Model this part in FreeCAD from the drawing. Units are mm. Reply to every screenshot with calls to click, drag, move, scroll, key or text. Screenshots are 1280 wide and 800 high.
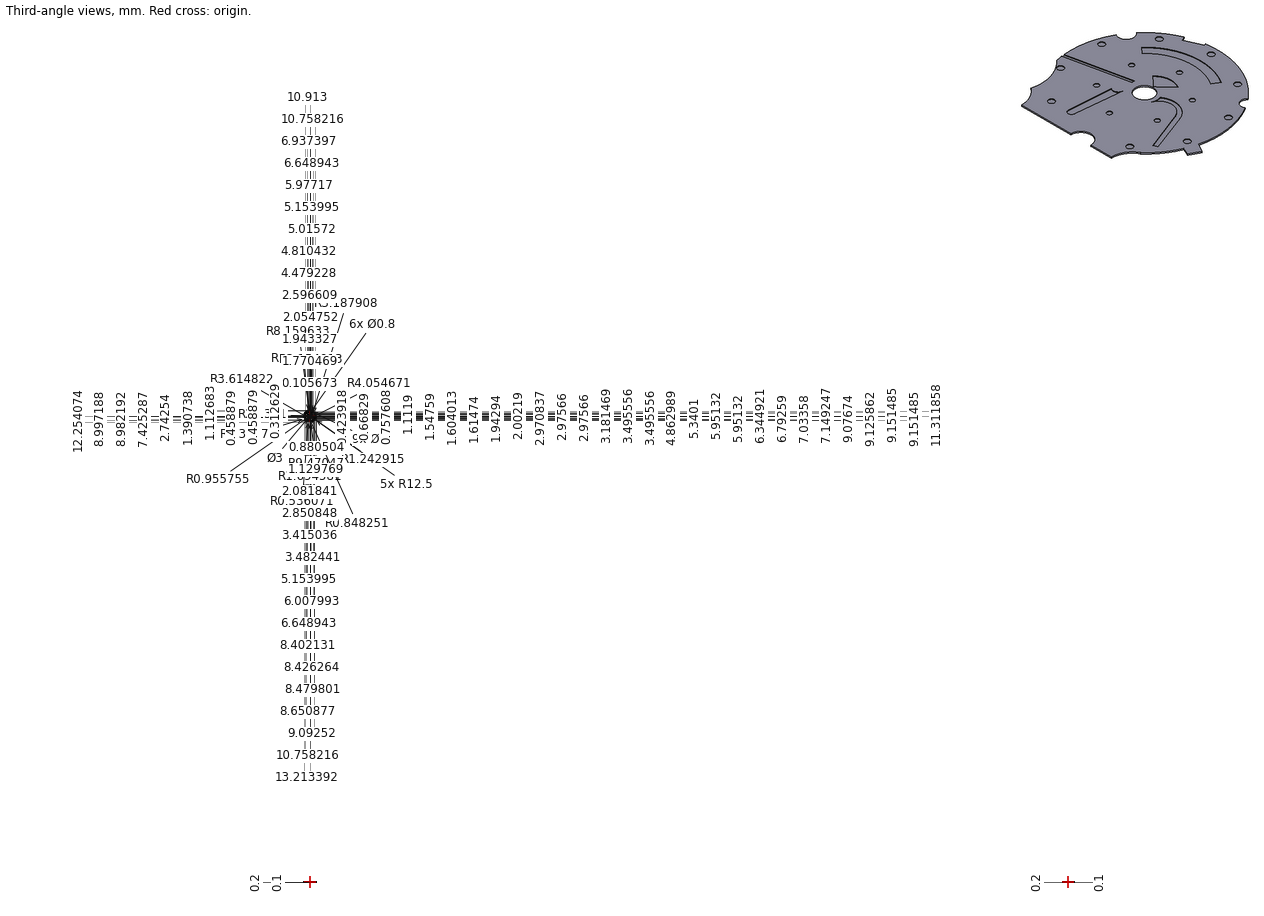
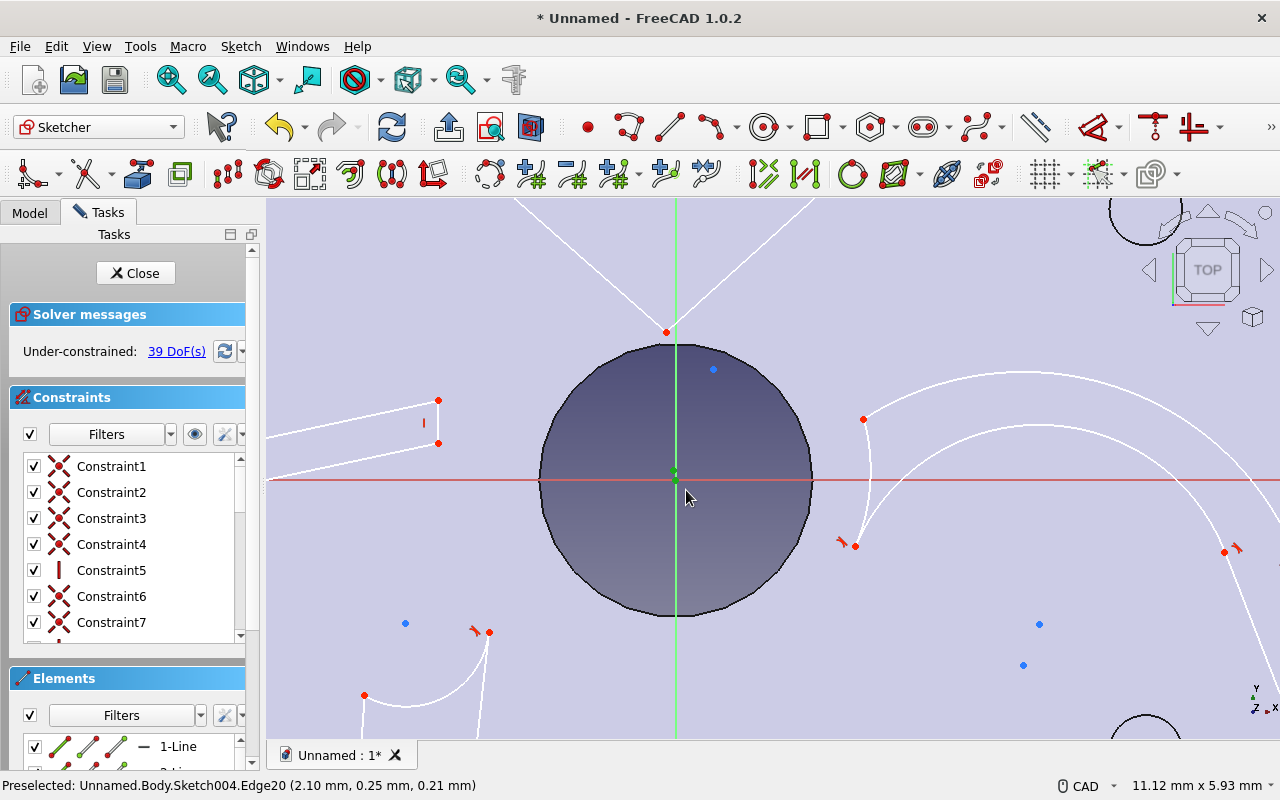
key(c)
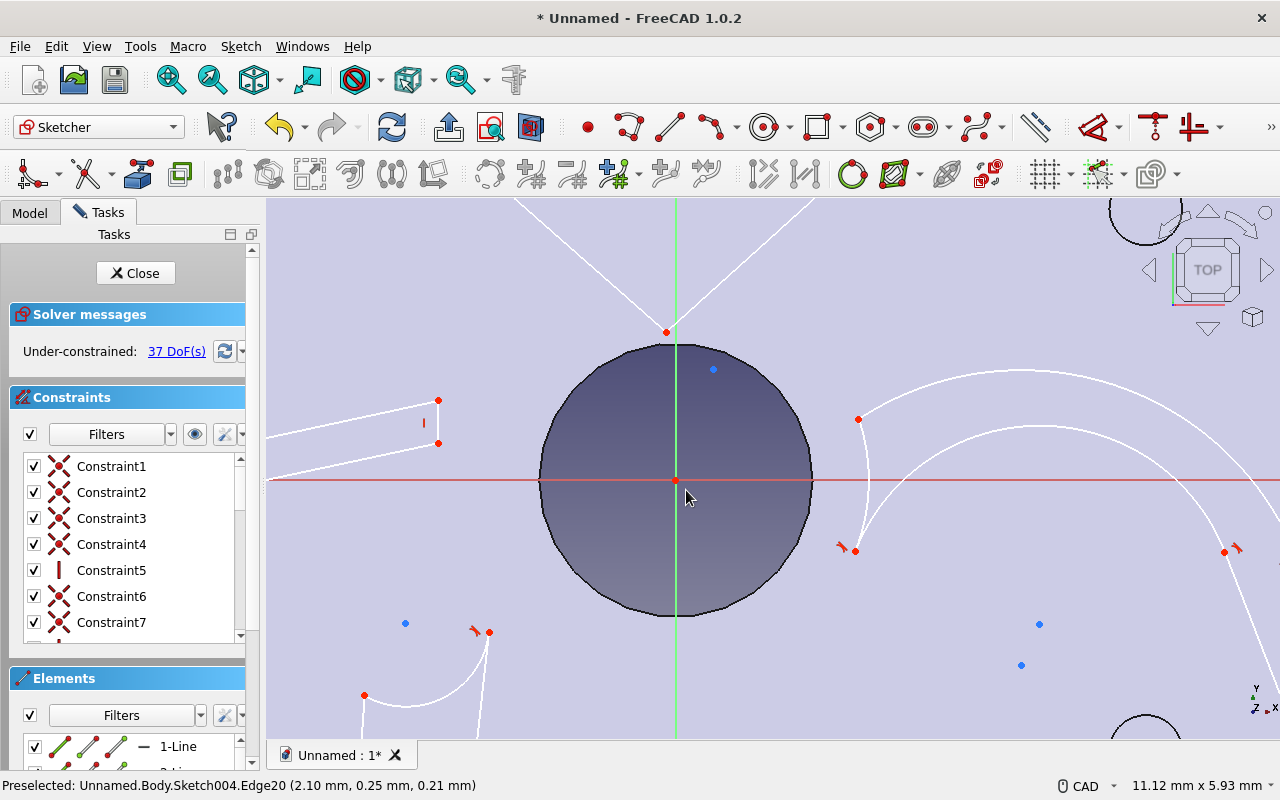
key(d)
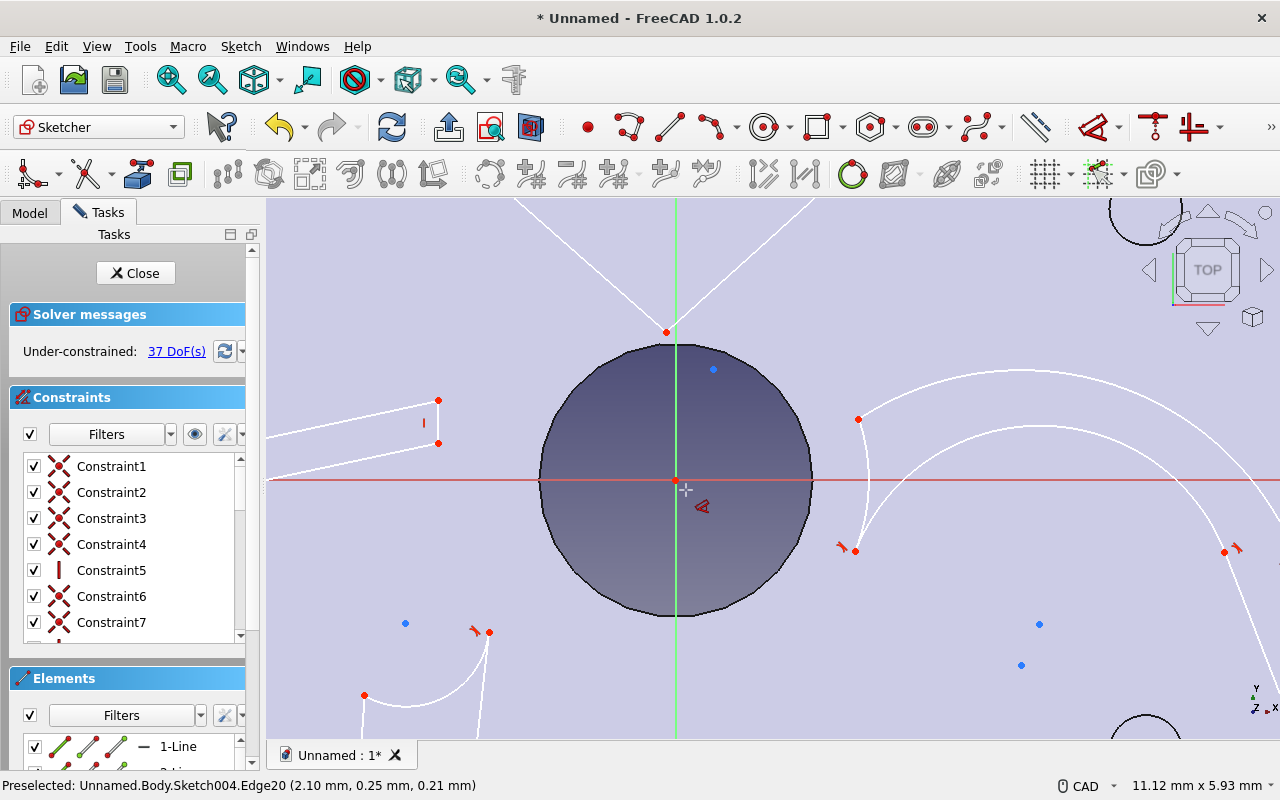
scroll(759, 463, down, 8)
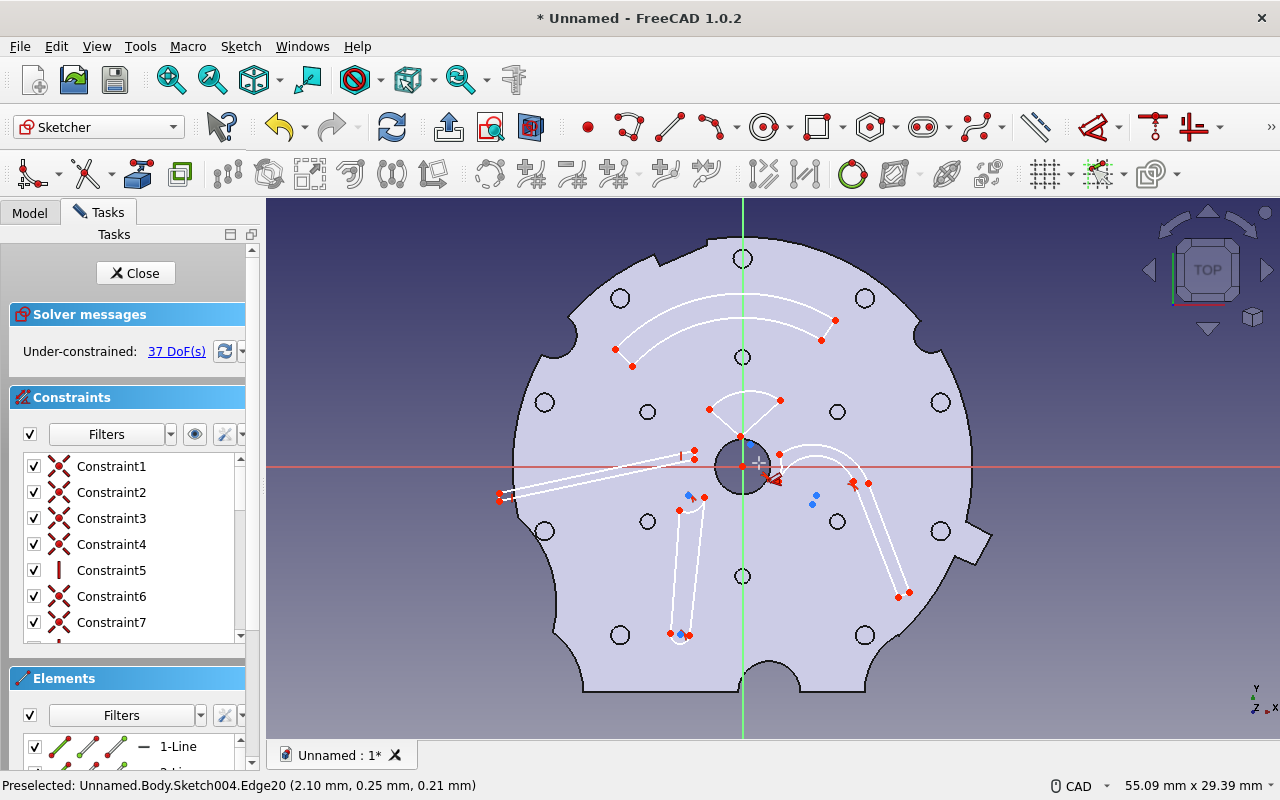
click(764, 319)
click(851, 322)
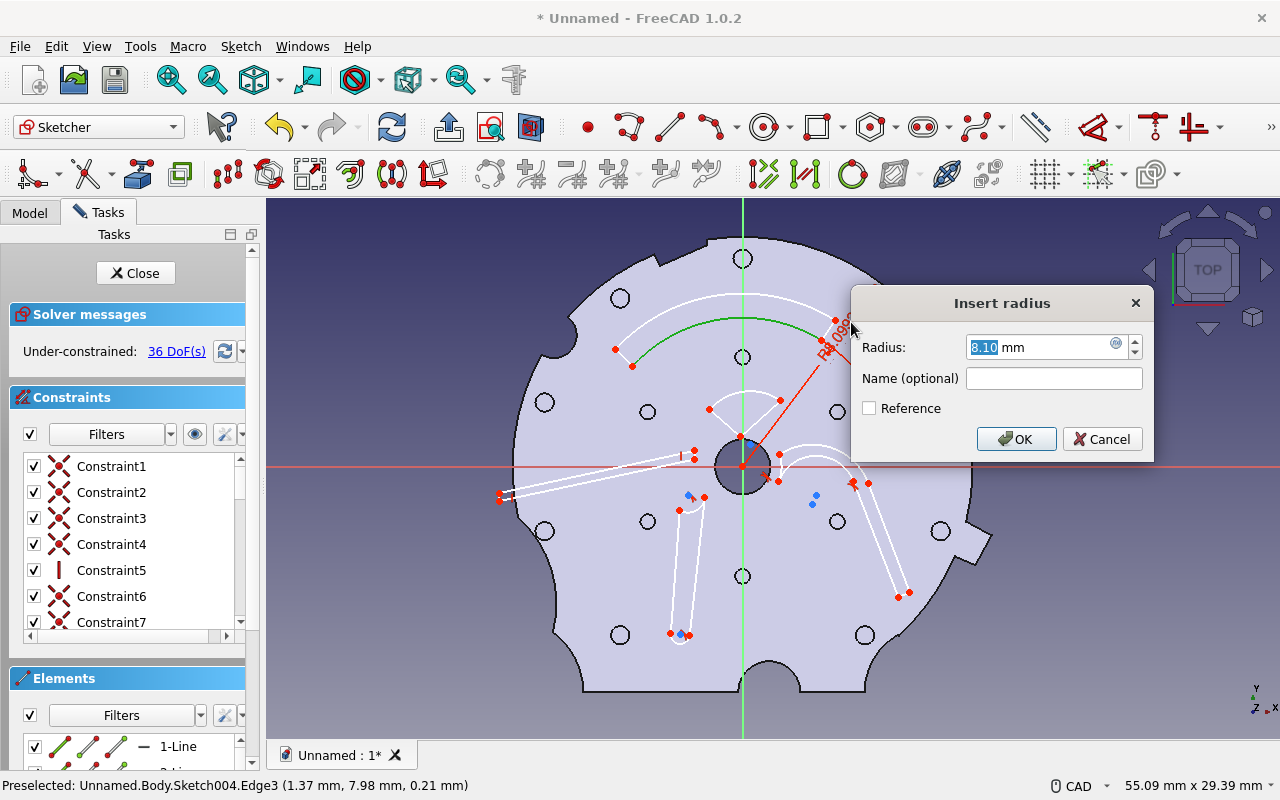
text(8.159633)
key(Return)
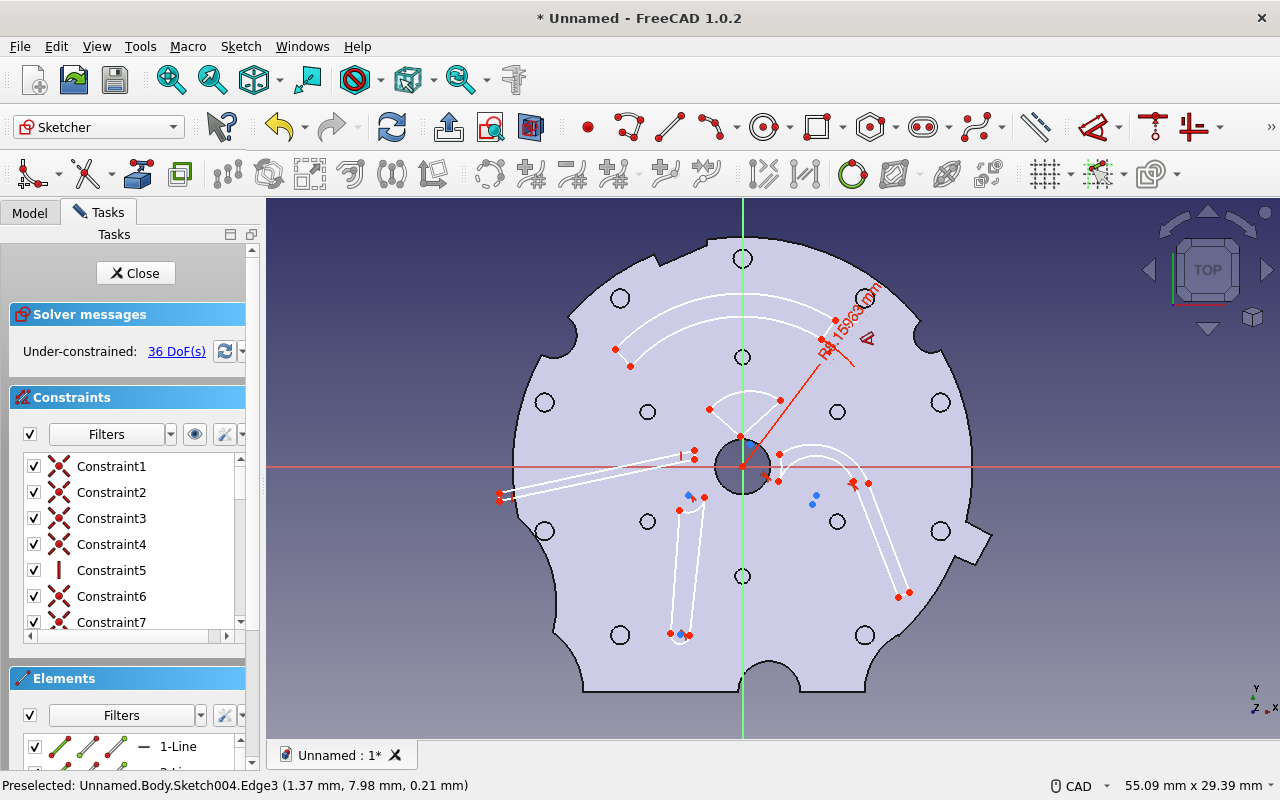
click(768, 295)
click(773, 263)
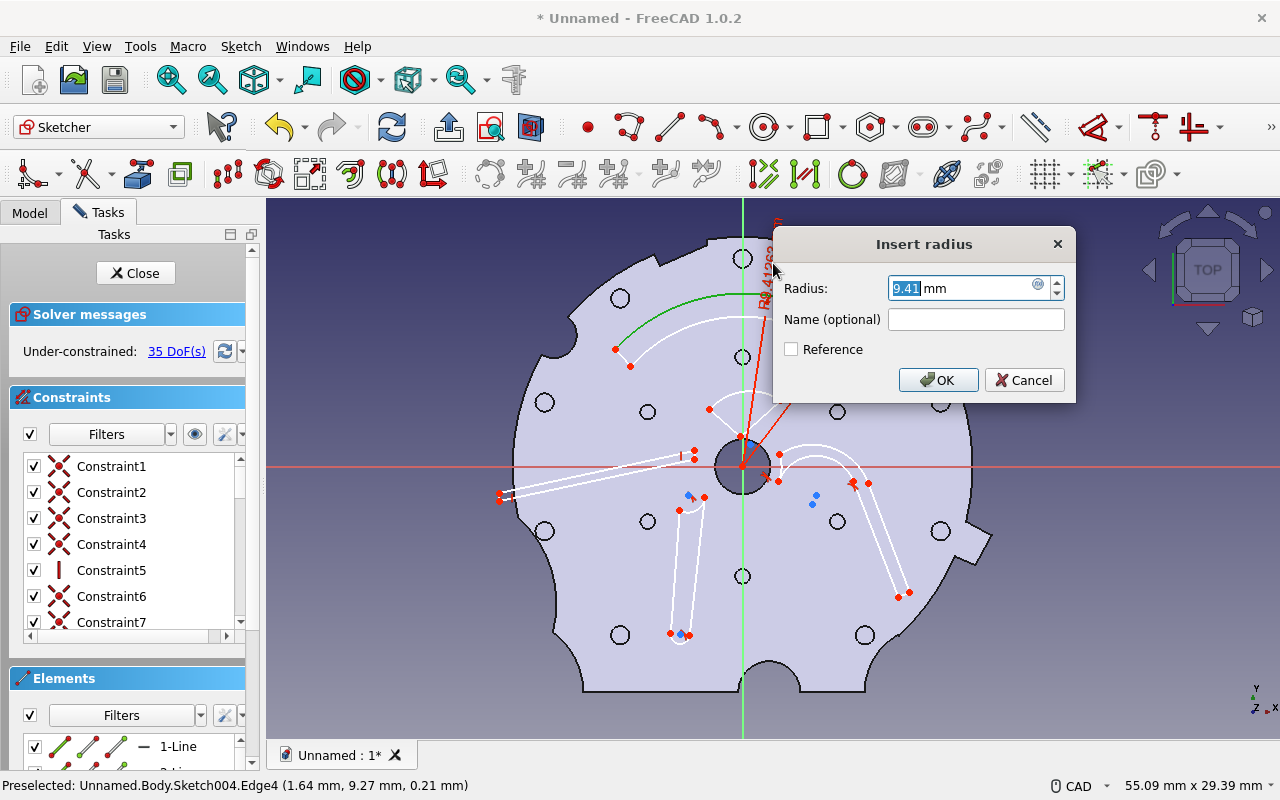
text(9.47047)
key(Return)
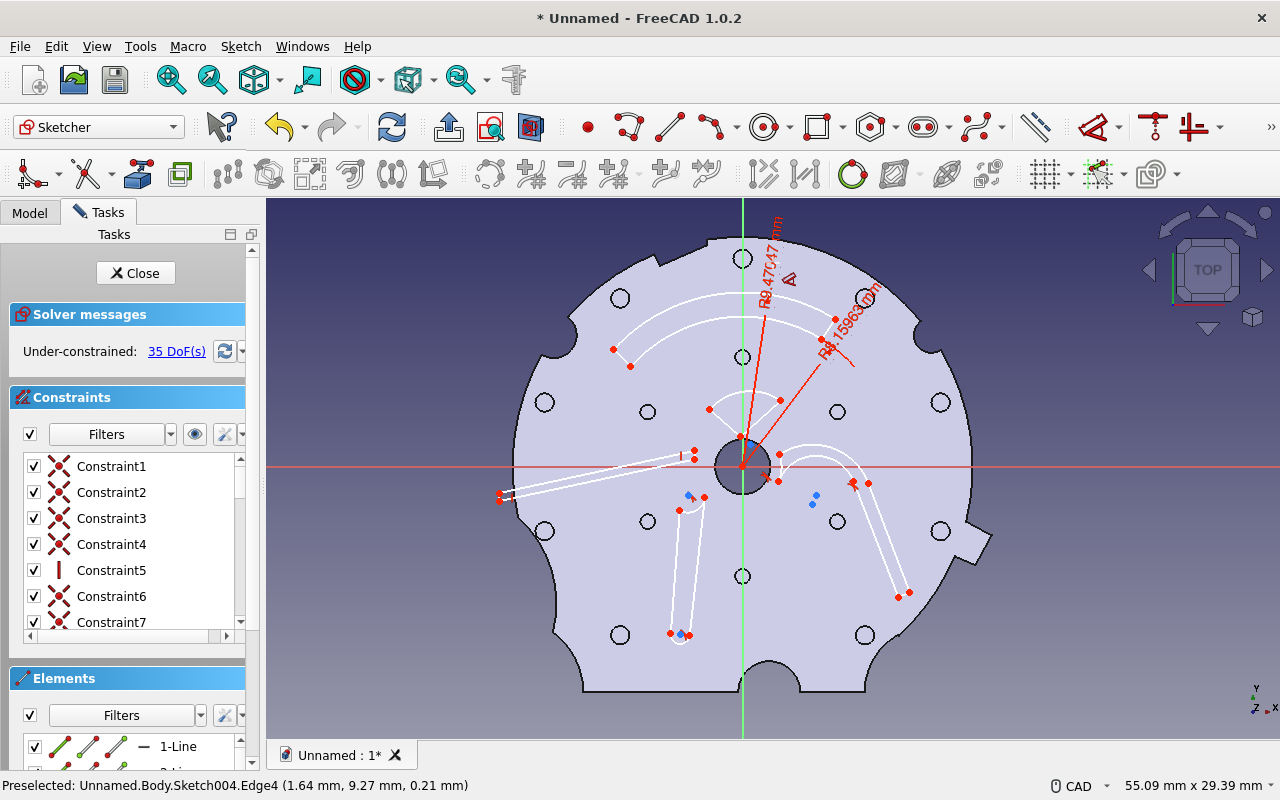
scroll(689, 513, up, 5)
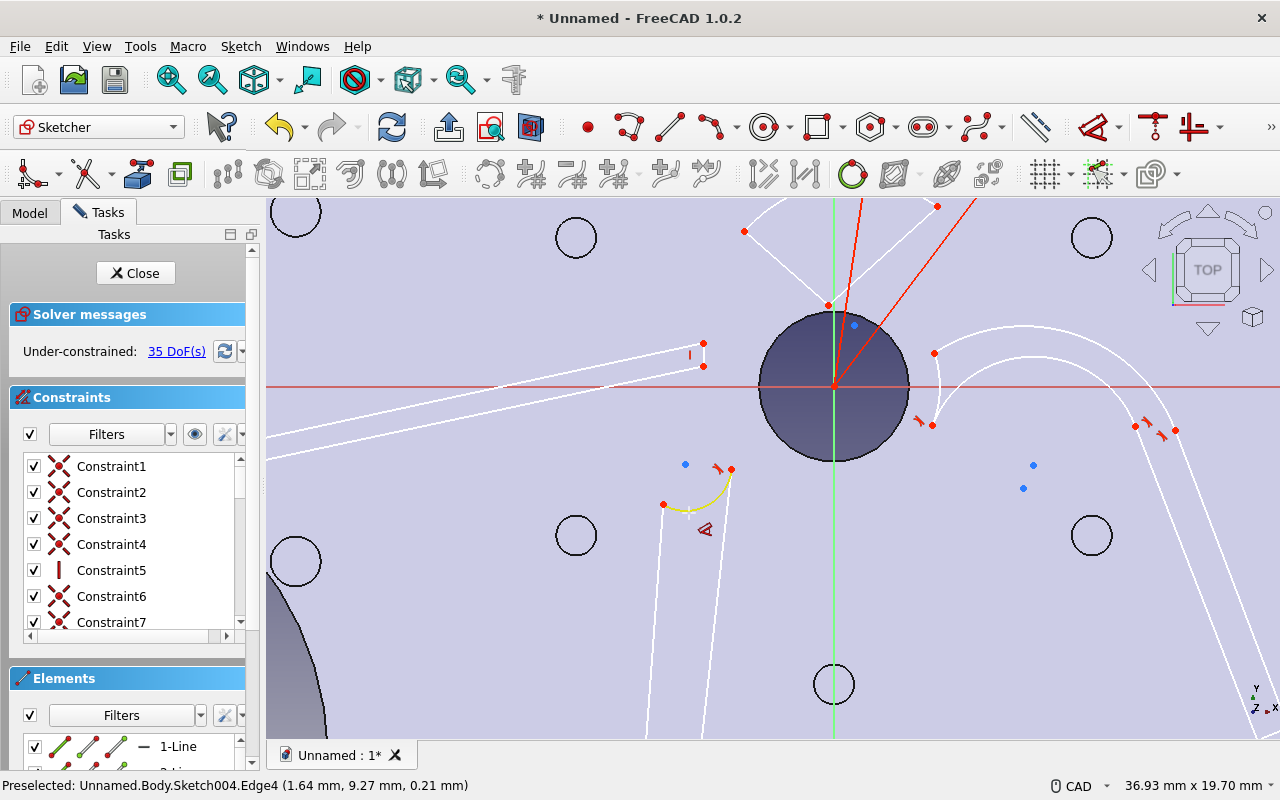
click(689, 511)
click(691, 543)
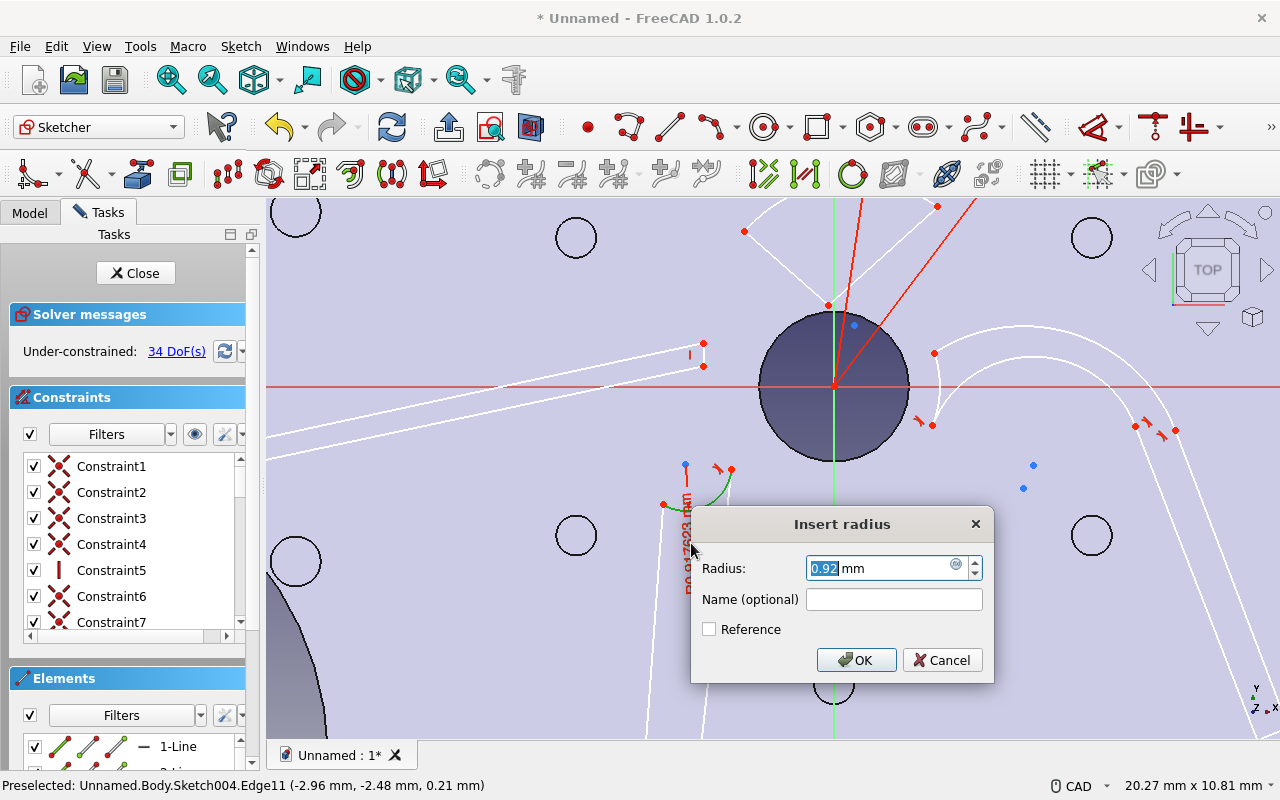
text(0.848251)
key(Return)